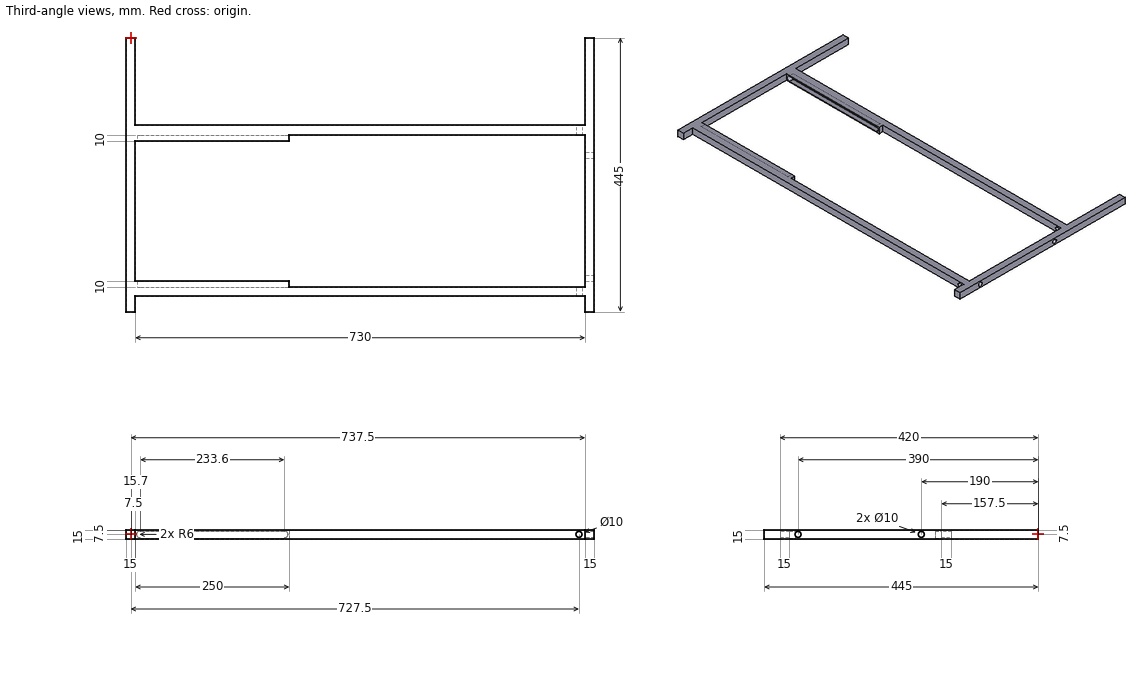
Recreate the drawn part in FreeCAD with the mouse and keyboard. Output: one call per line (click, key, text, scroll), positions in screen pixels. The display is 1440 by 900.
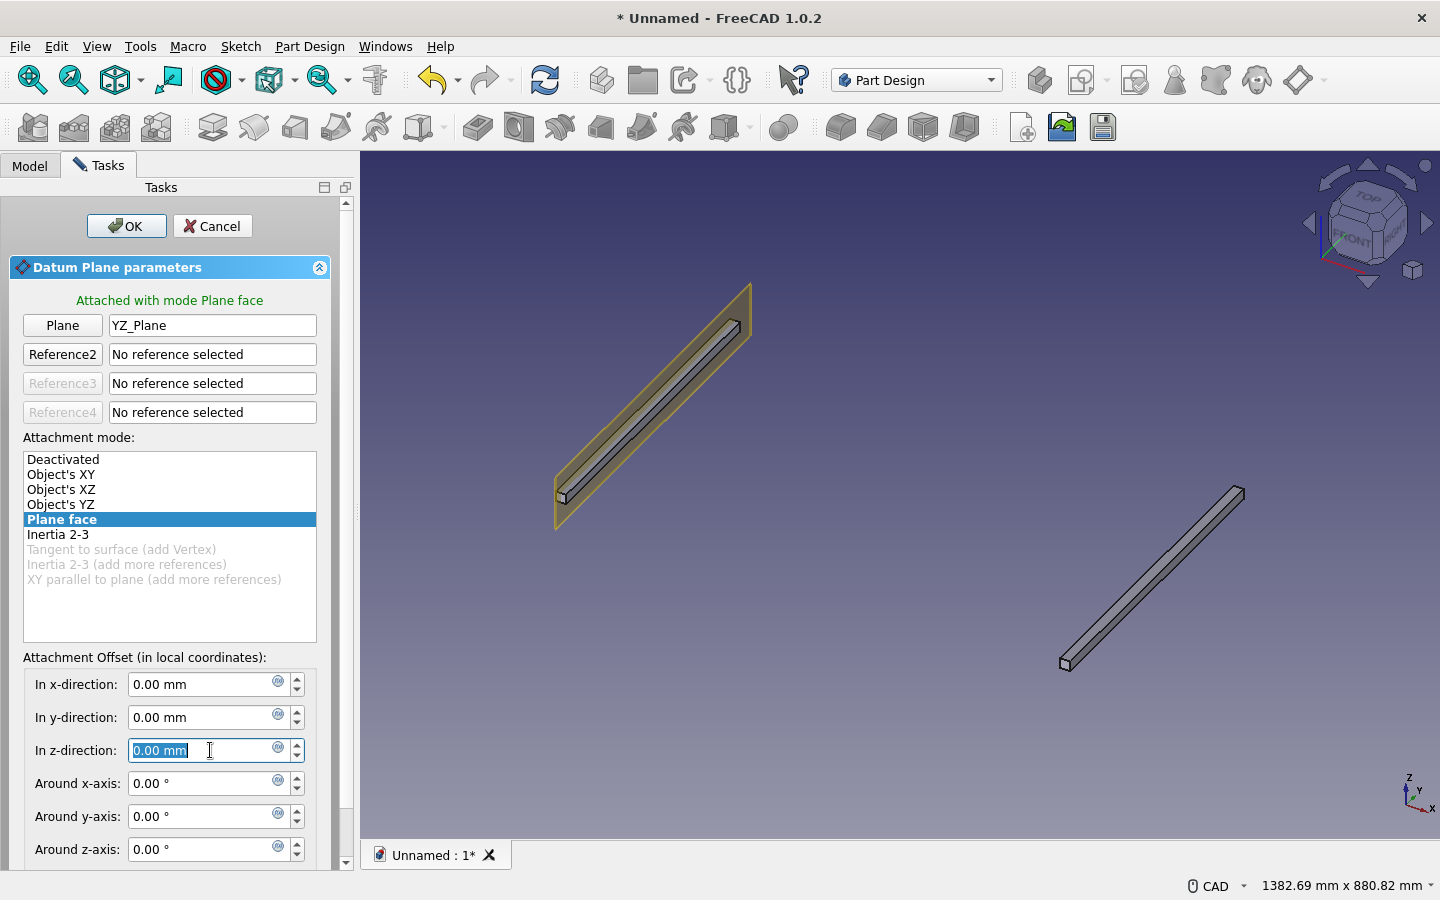
text(7.5)
key(Tab)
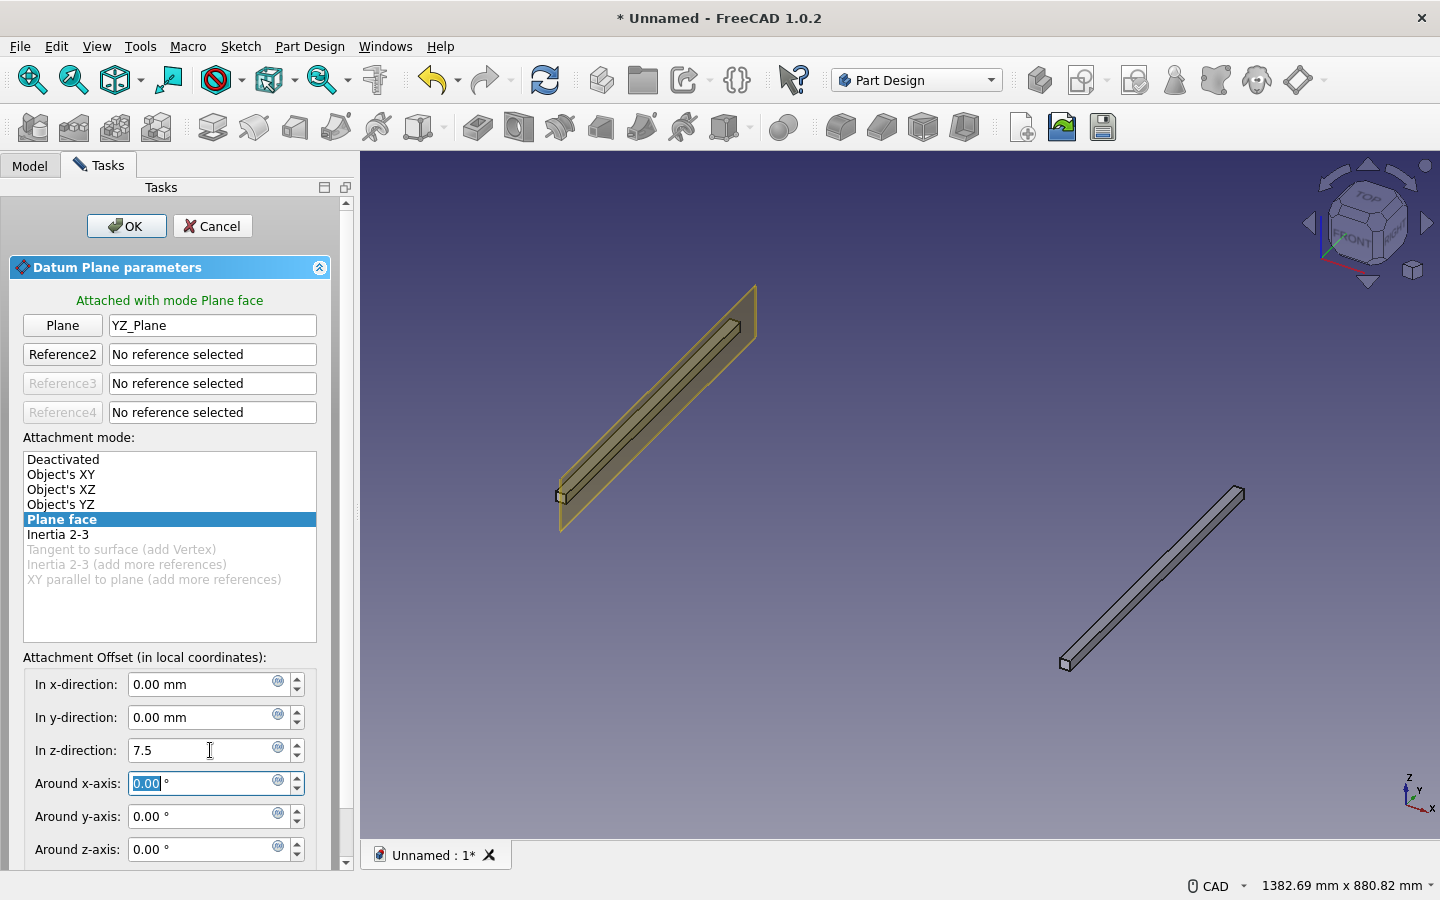
click(127, 226)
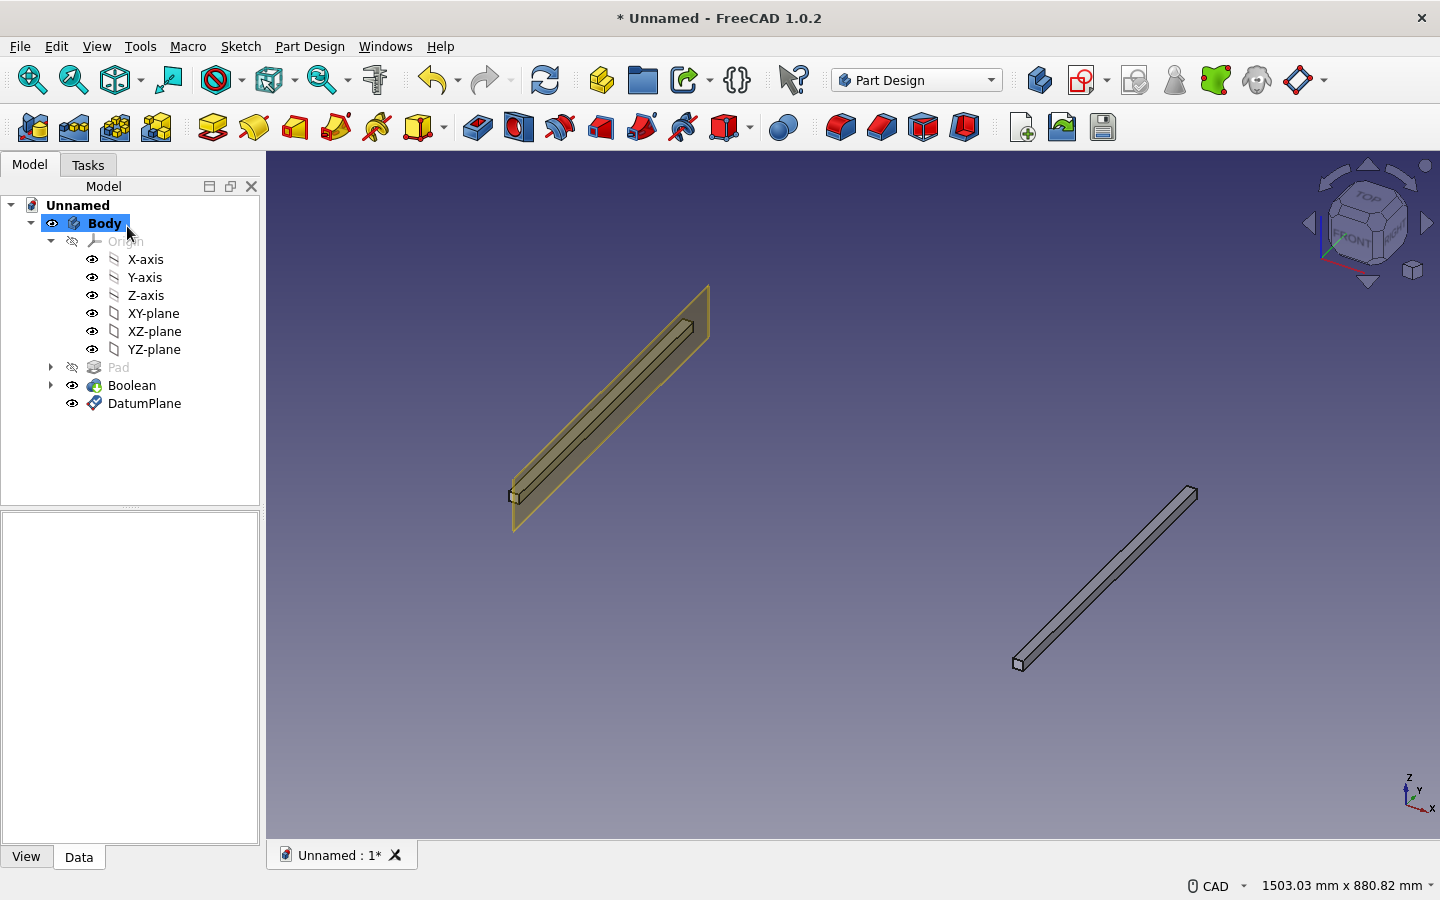
click(117, 403)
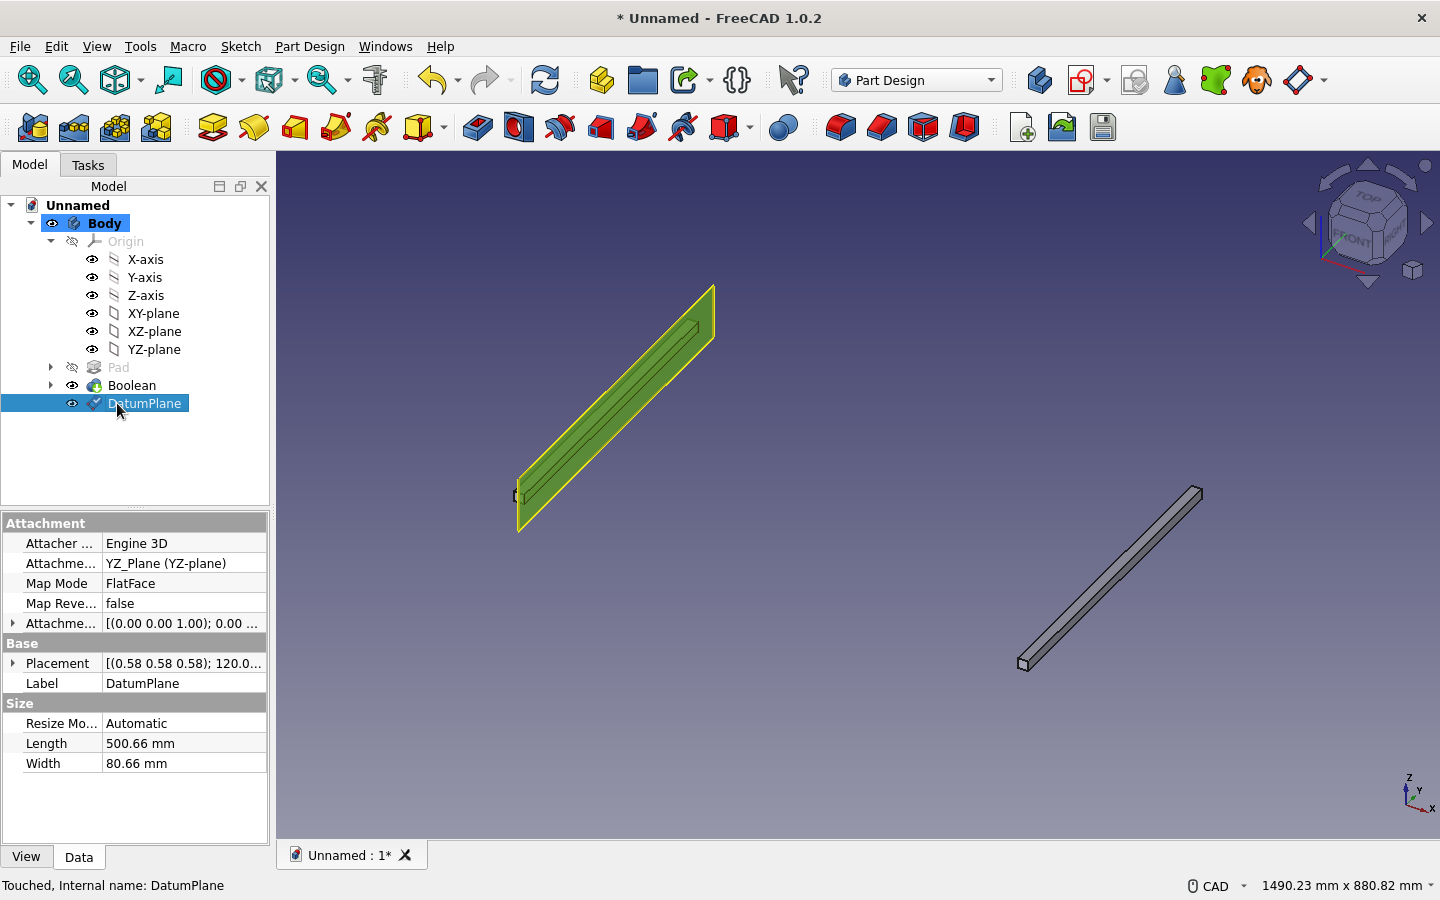
click(1080, 80)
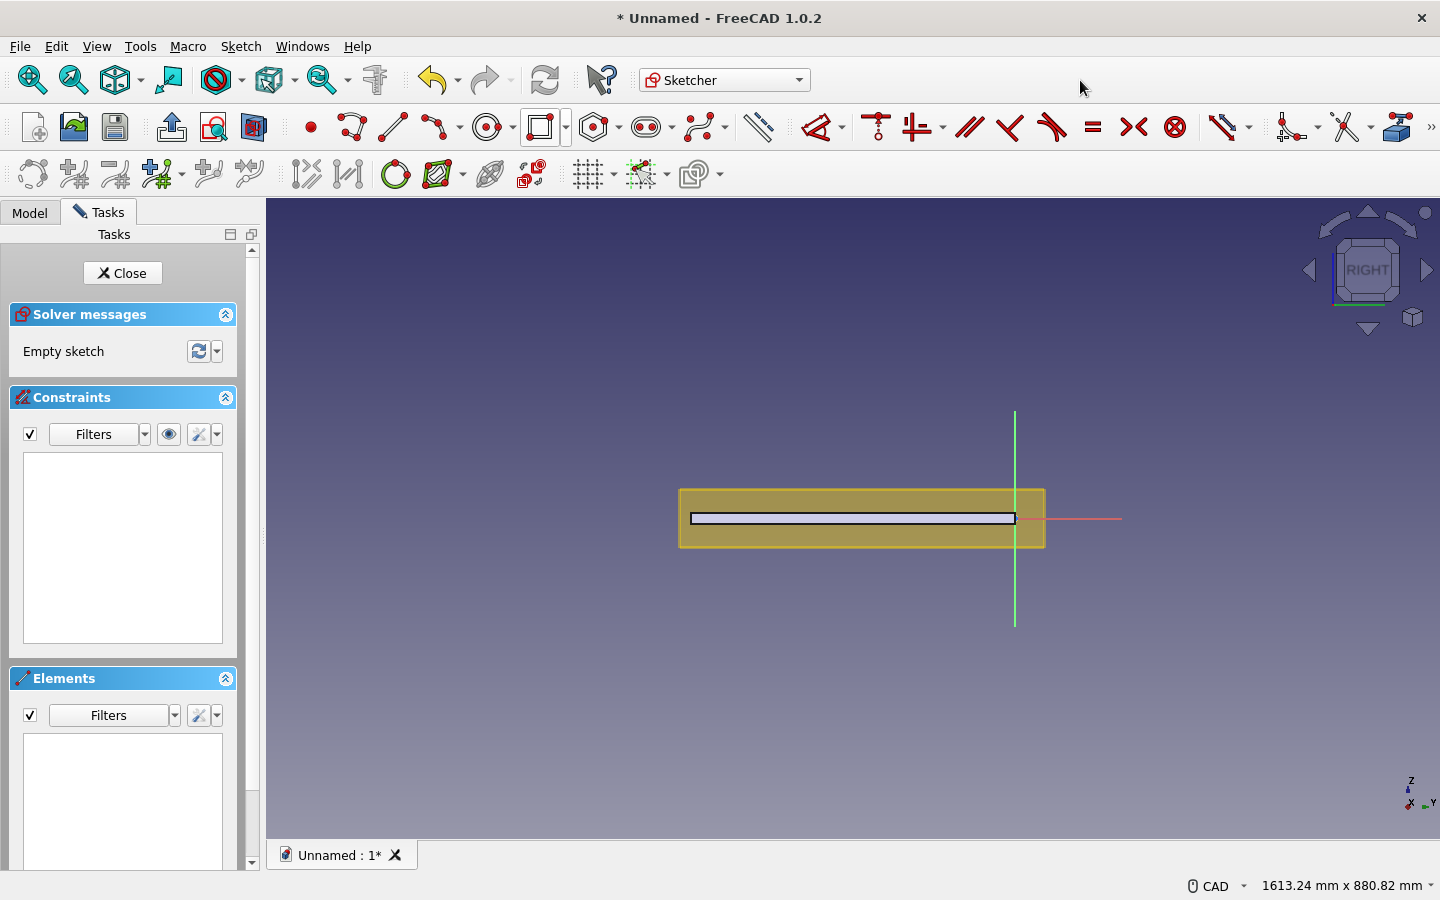
click(254, 128)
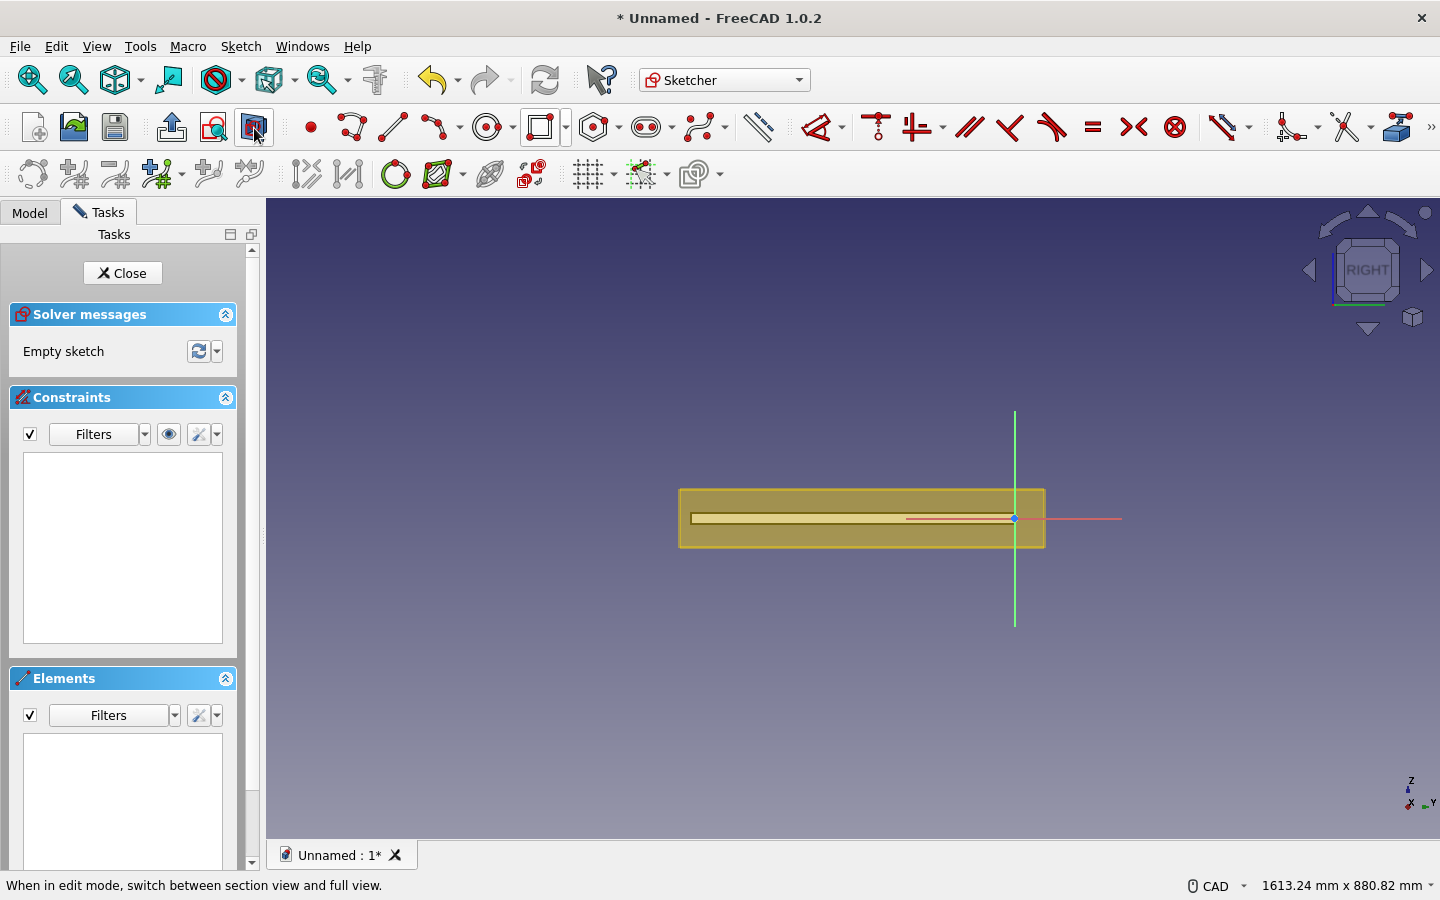
scroll(925, 518, up, 4)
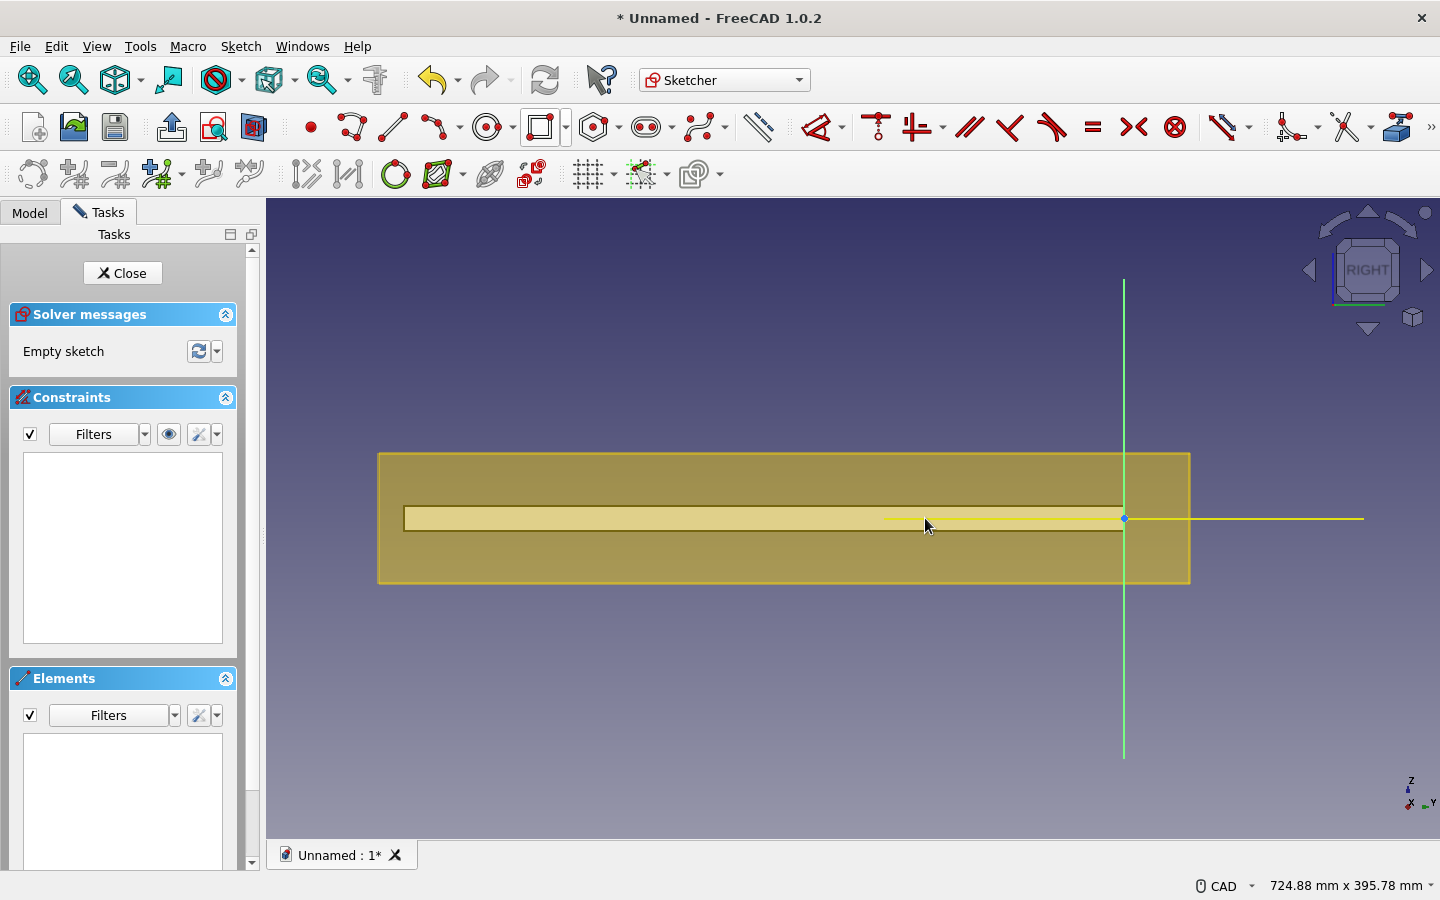
click(540, 128)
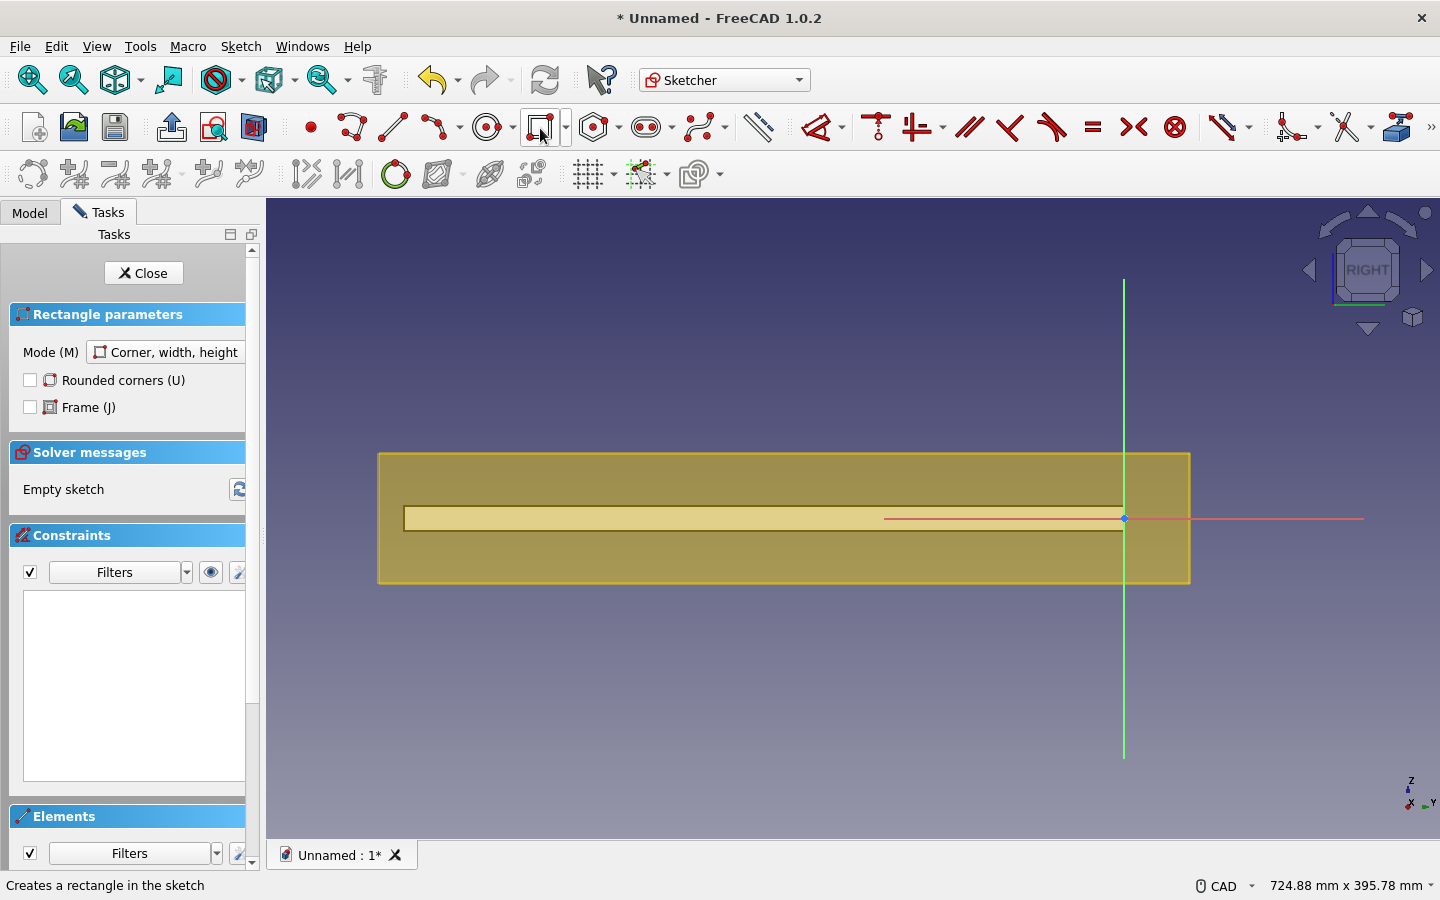
scroll(444, 506, up, 2)